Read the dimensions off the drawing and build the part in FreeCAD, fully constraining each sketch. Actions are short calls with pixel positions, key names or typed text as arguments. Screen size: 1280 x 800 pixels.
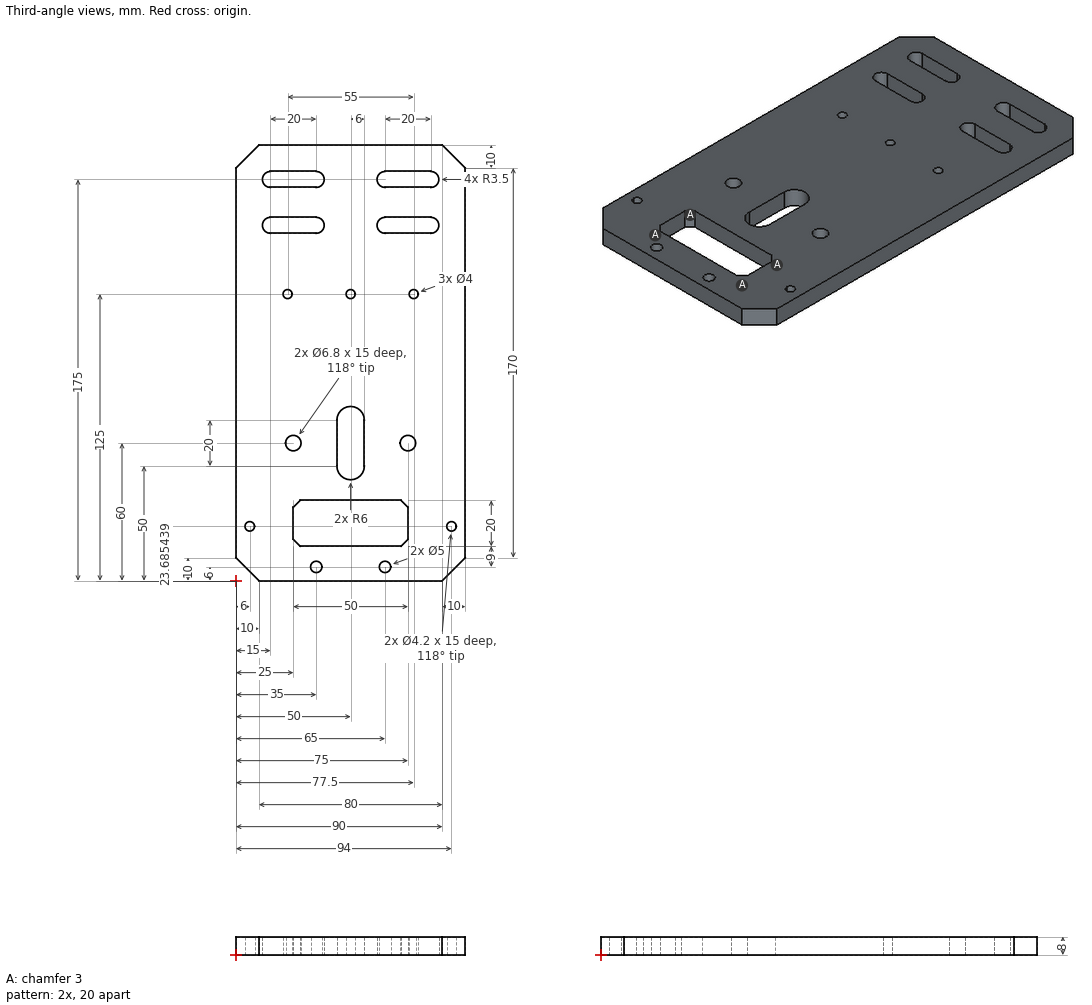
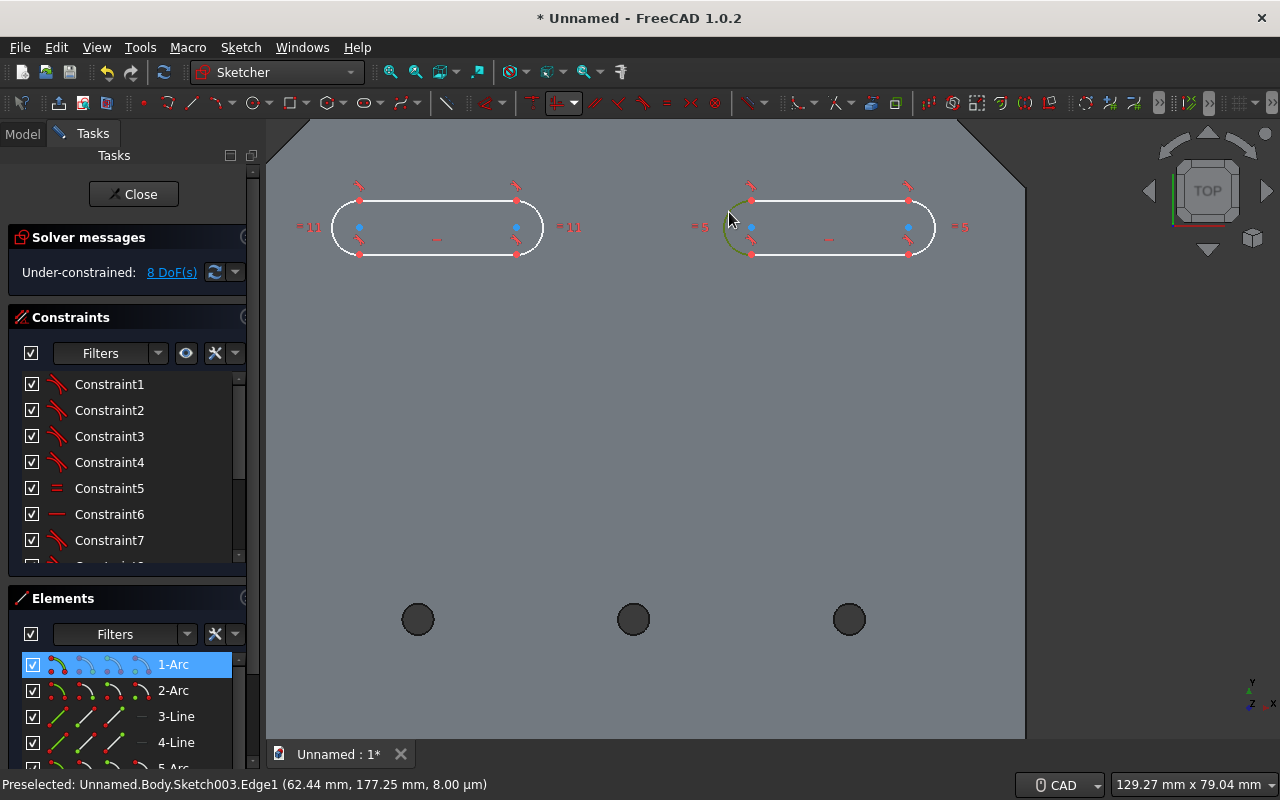
click(337, 212)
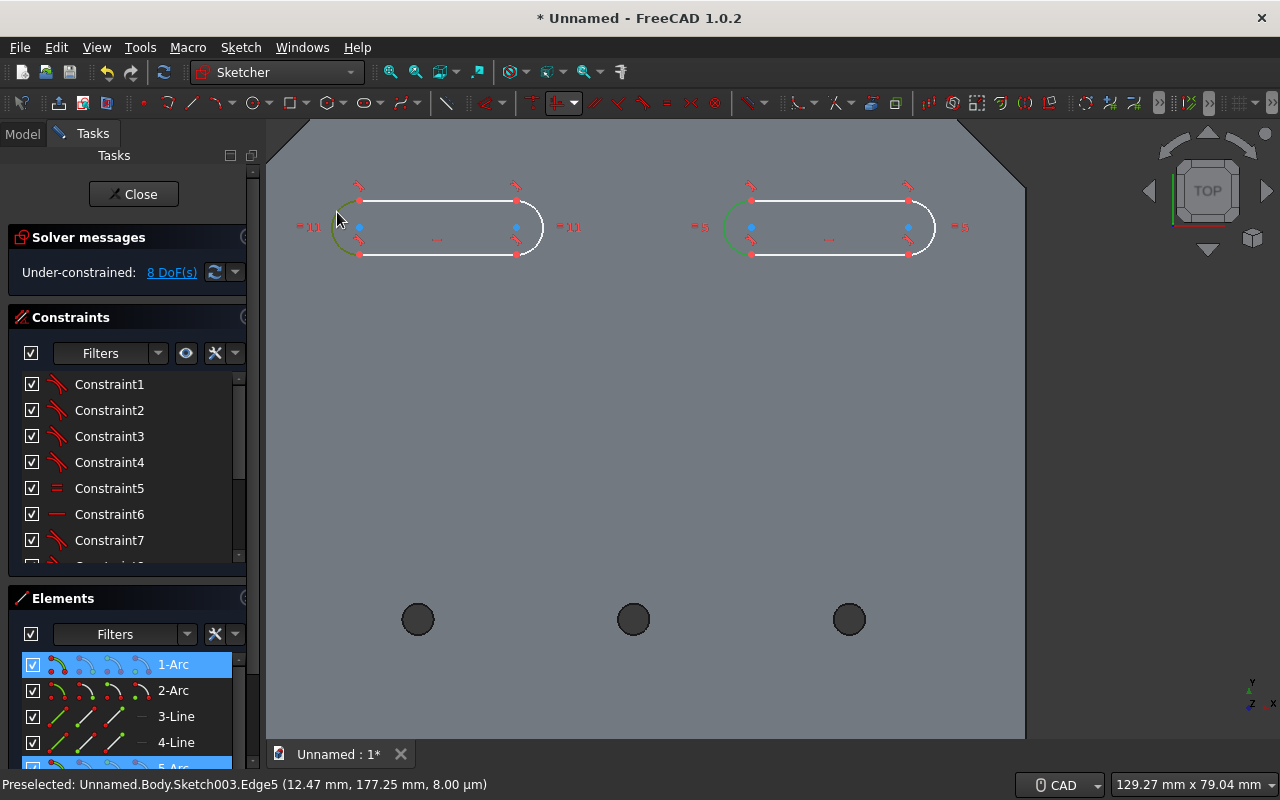
click(668, 104)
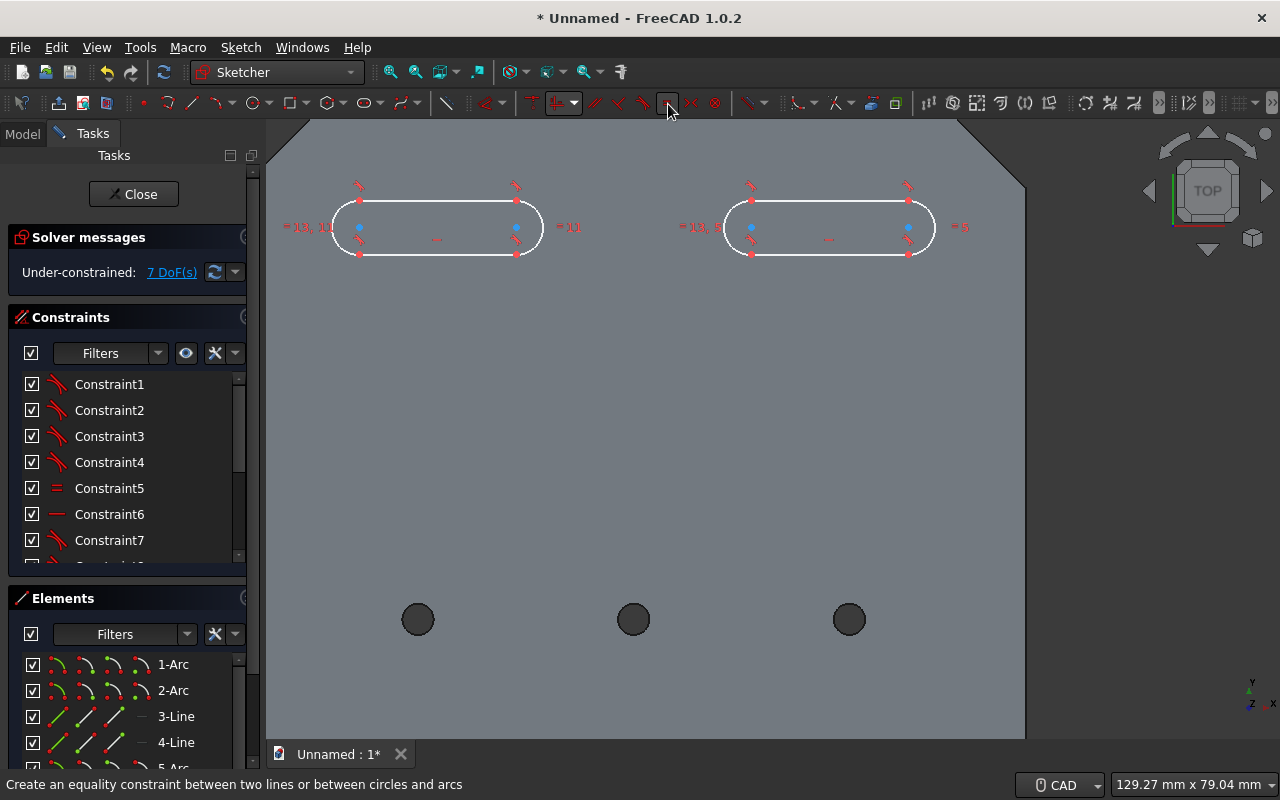
click(486, 104)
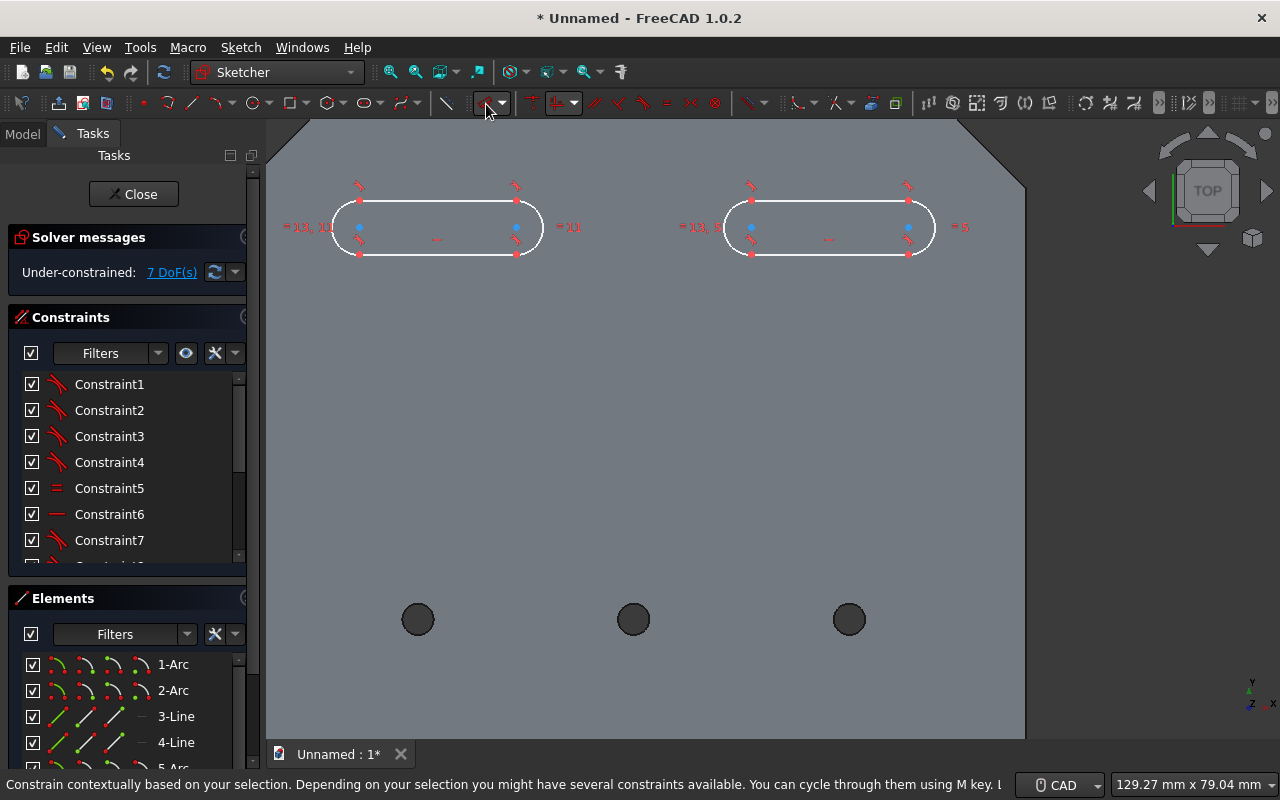
scroll(729, 212, up, 2)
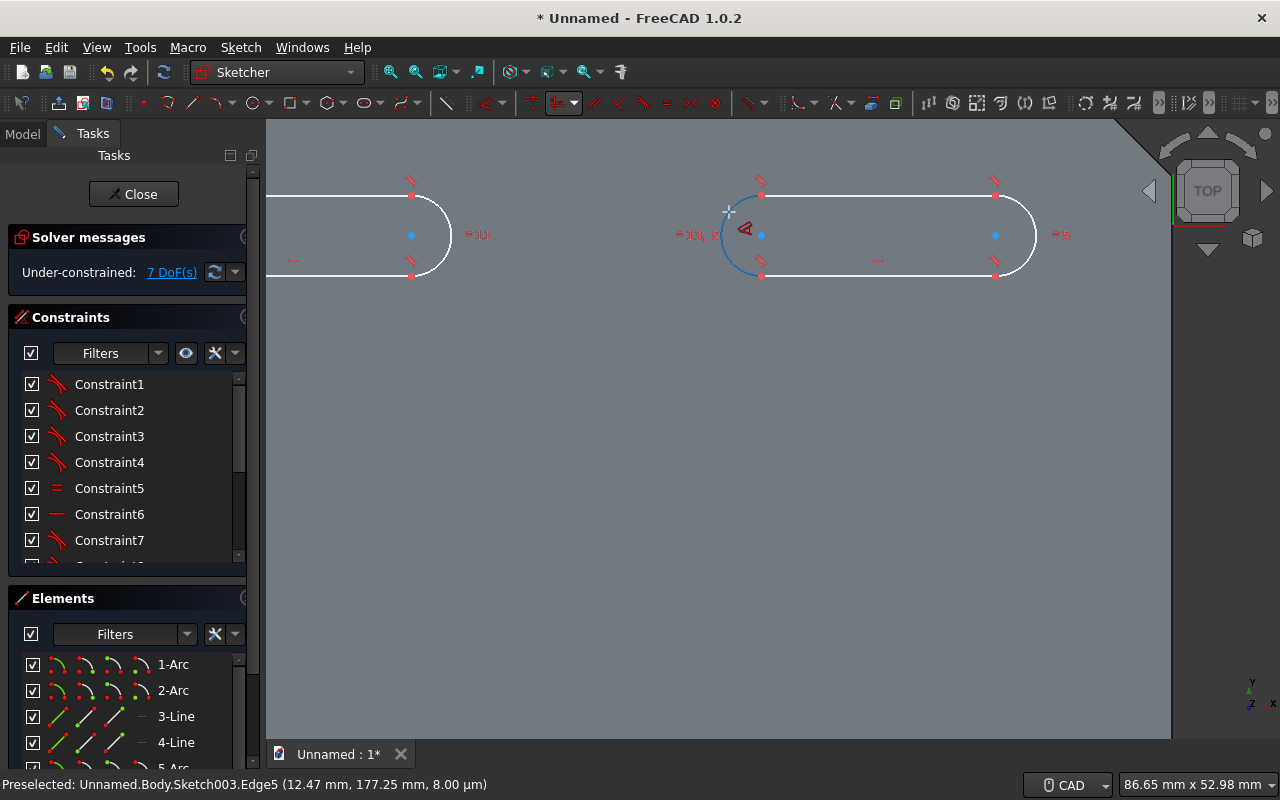
click(729, 212)
click(703, 193)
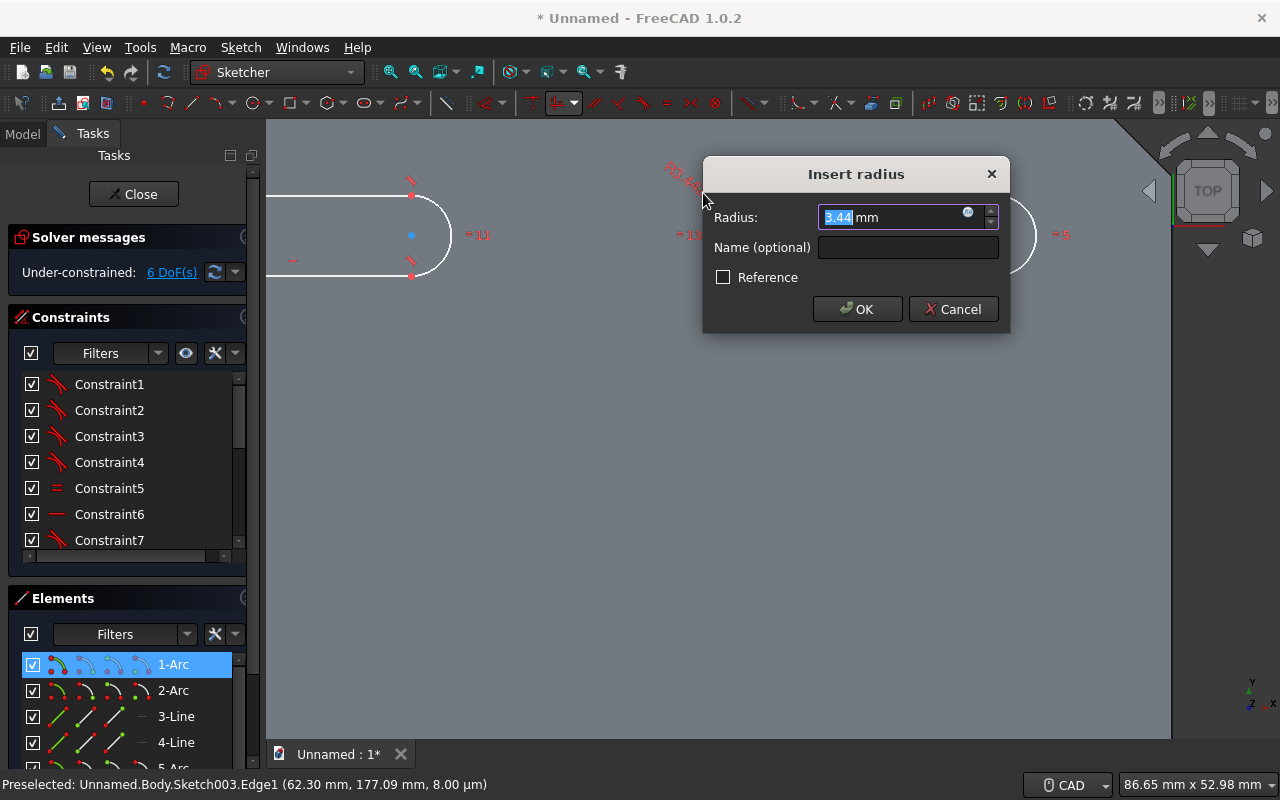
text(3.5)
key(Return)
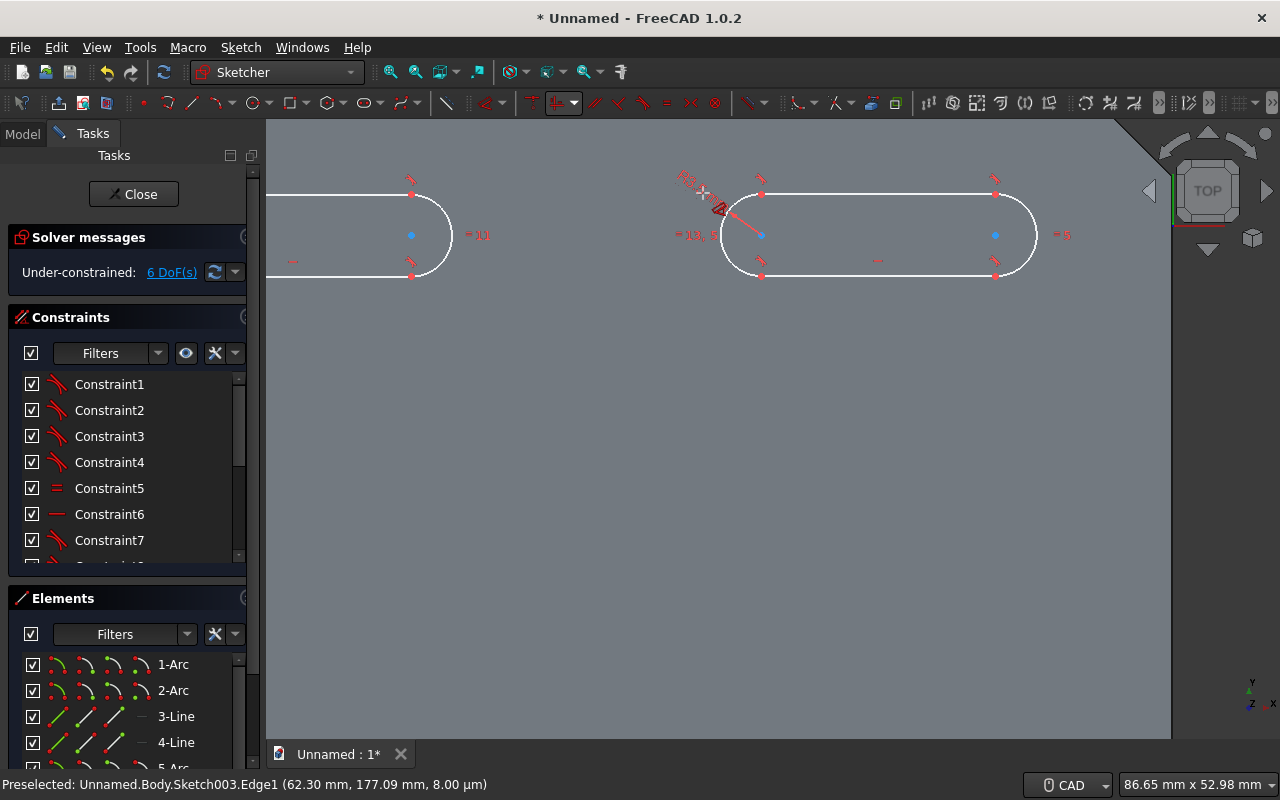
scroll(751, 224, down, 8)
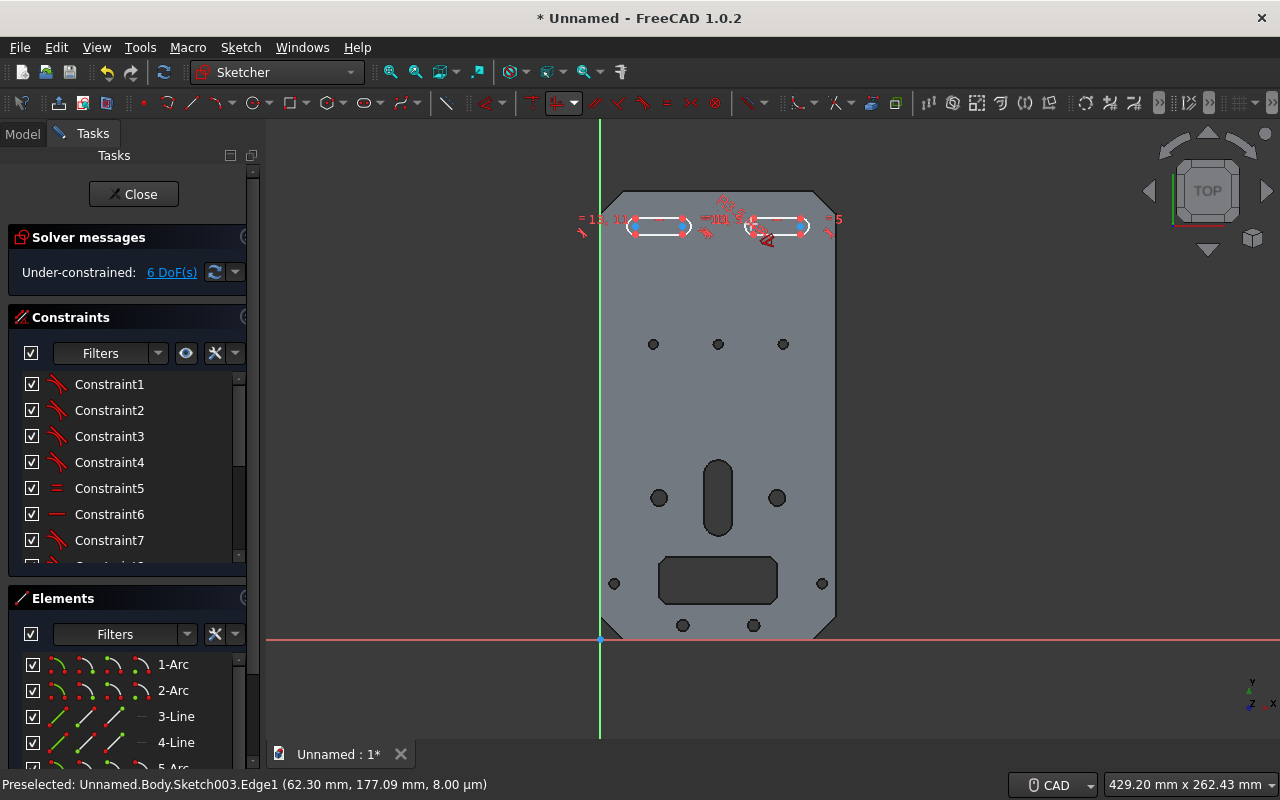
click(768, 218)
click(777, 184)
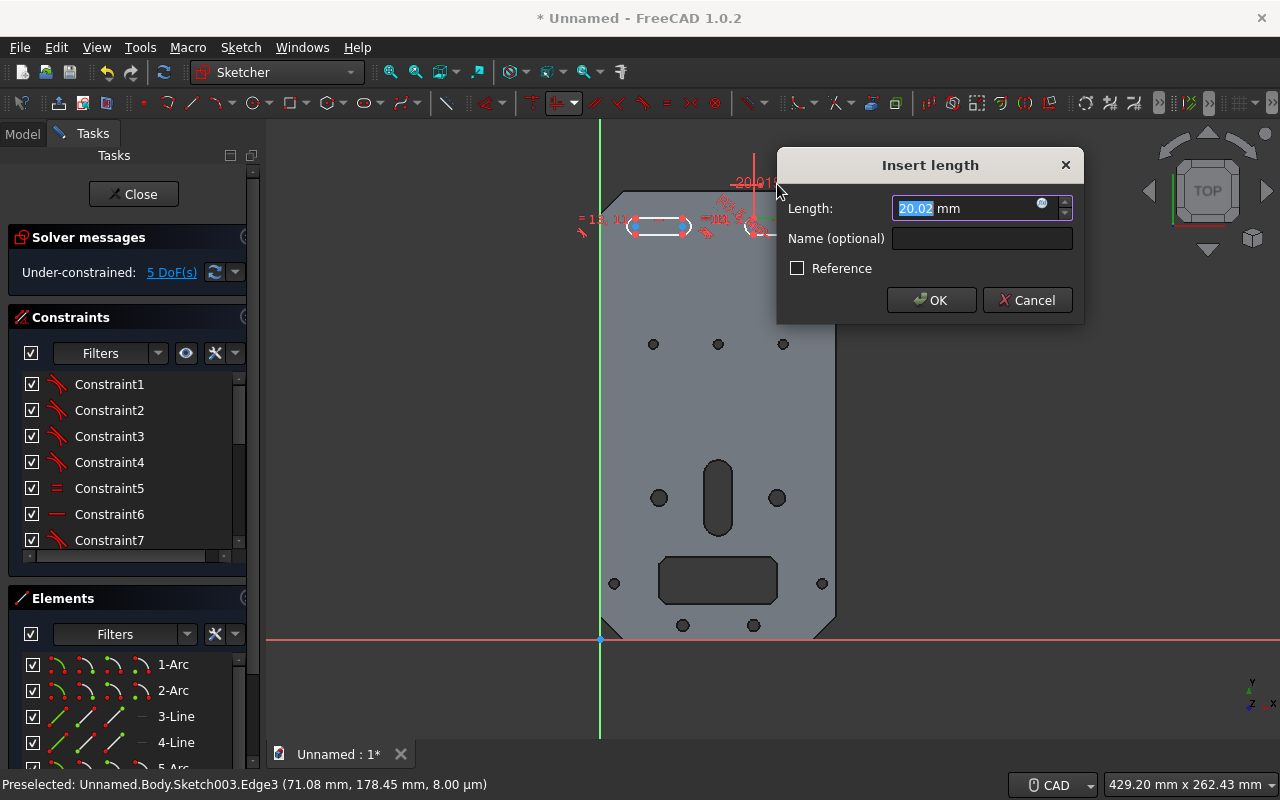
text(20)
key(Return)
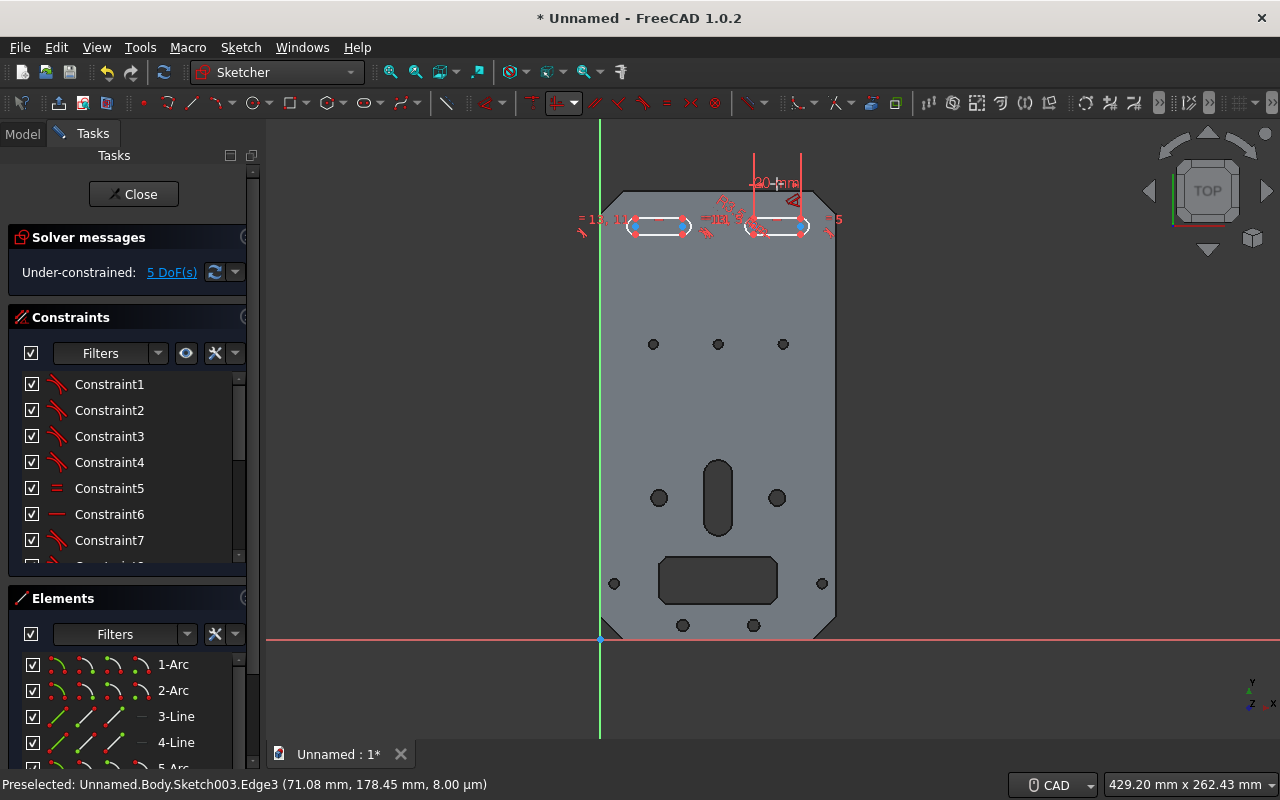
click(650, 218)
click(659, 184)